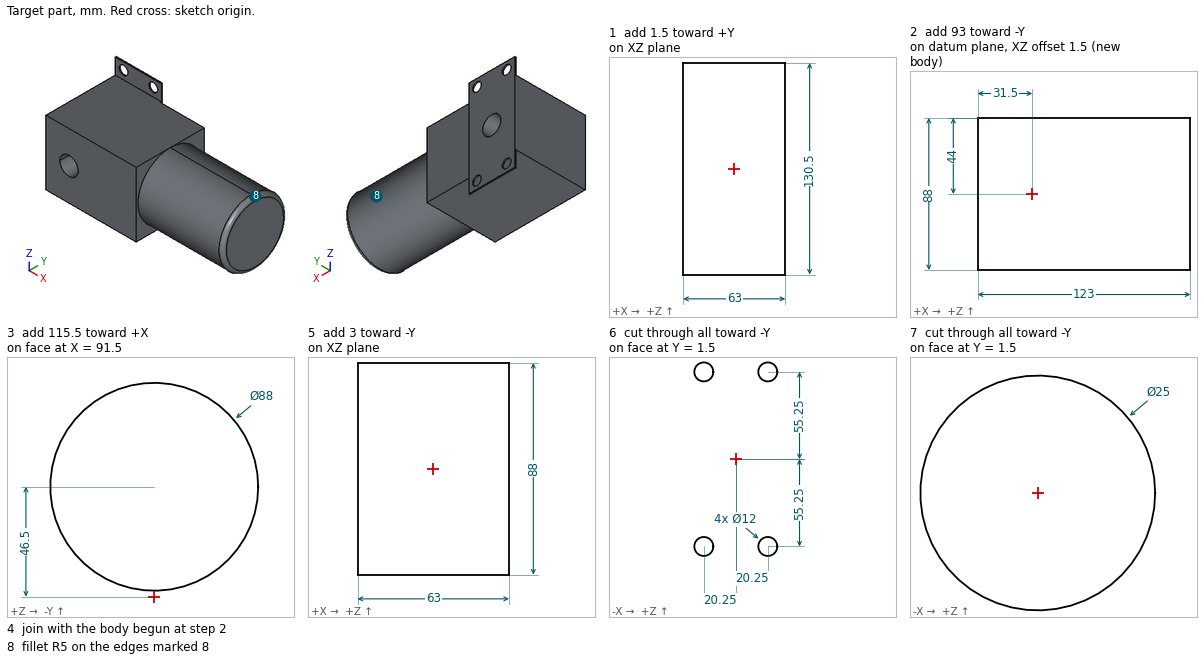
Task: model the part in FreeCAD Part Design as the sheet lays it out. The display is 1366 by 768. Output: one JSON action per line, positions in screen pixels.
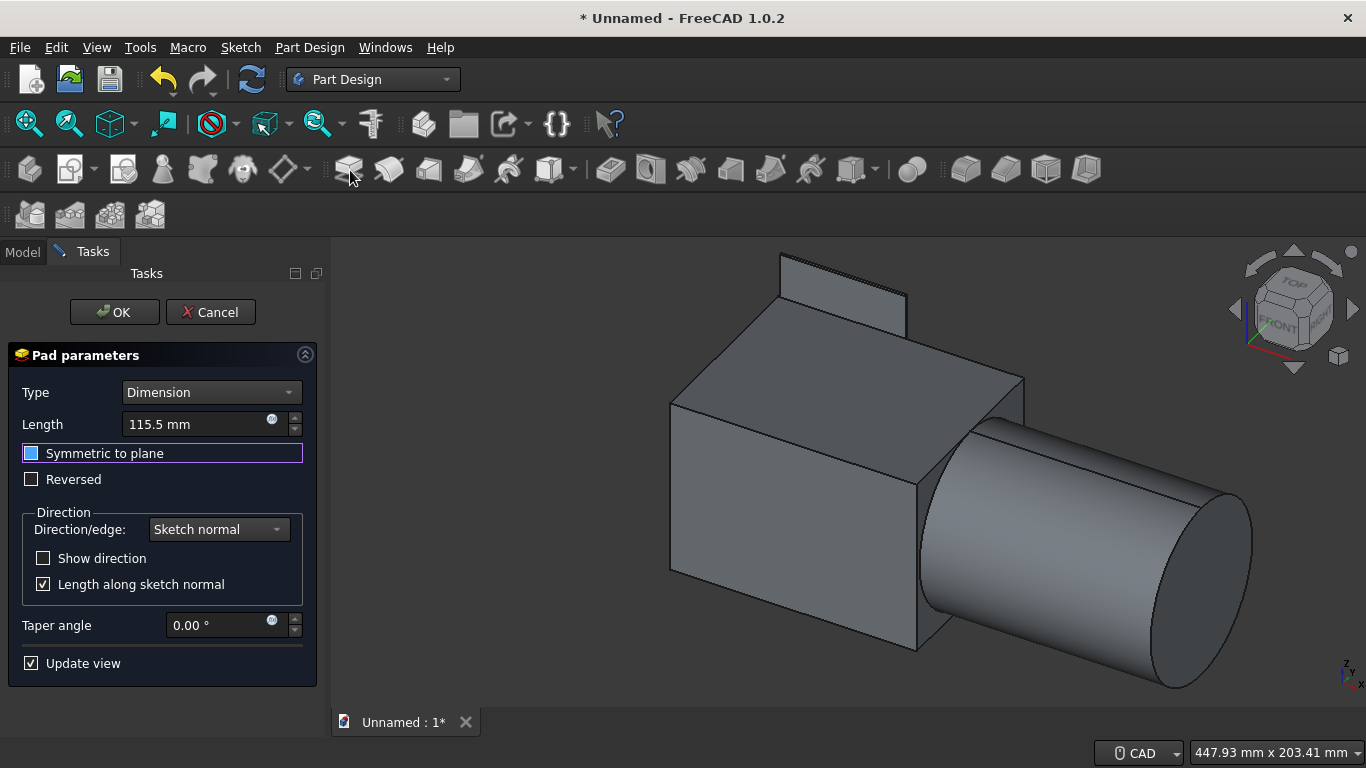
{"action": "left_click", "coordinate": [115, 312]}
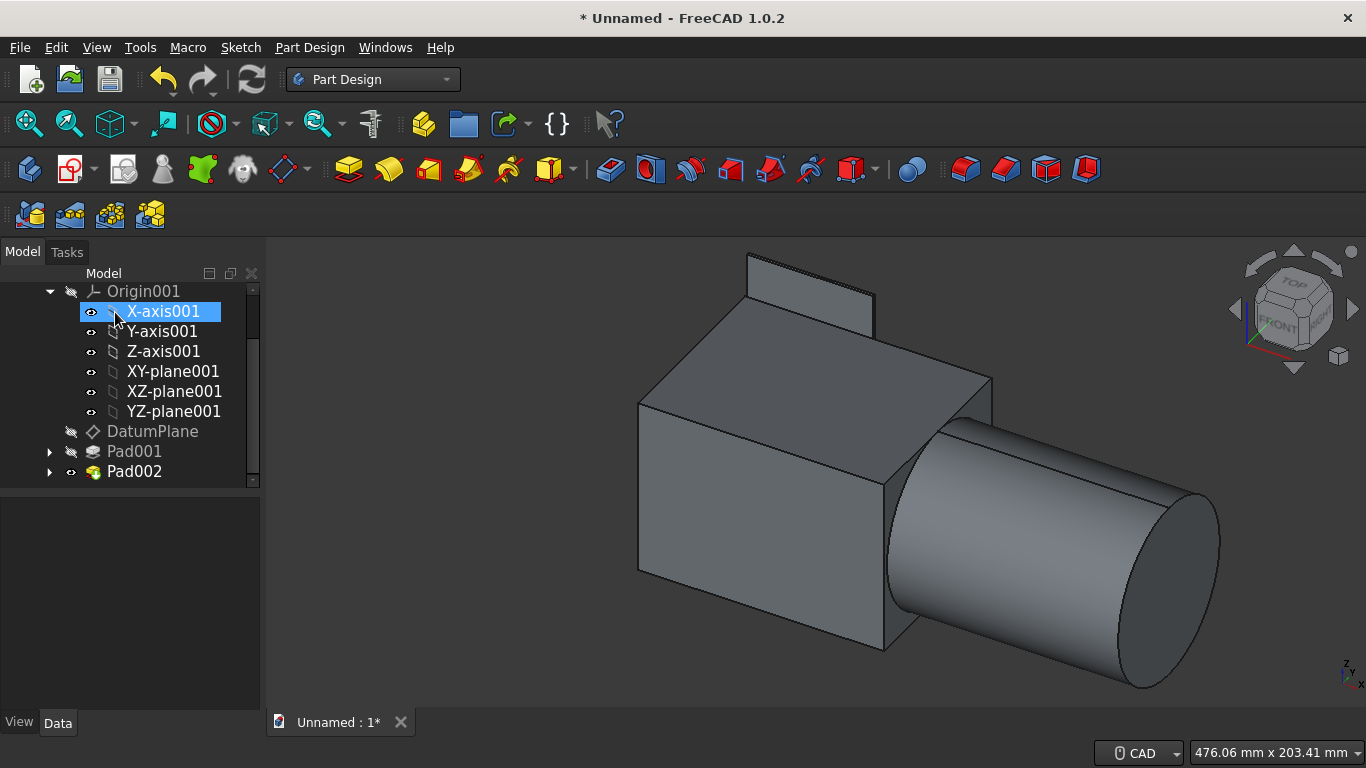
{"action": "left_click", "coordinate": [30, 124]}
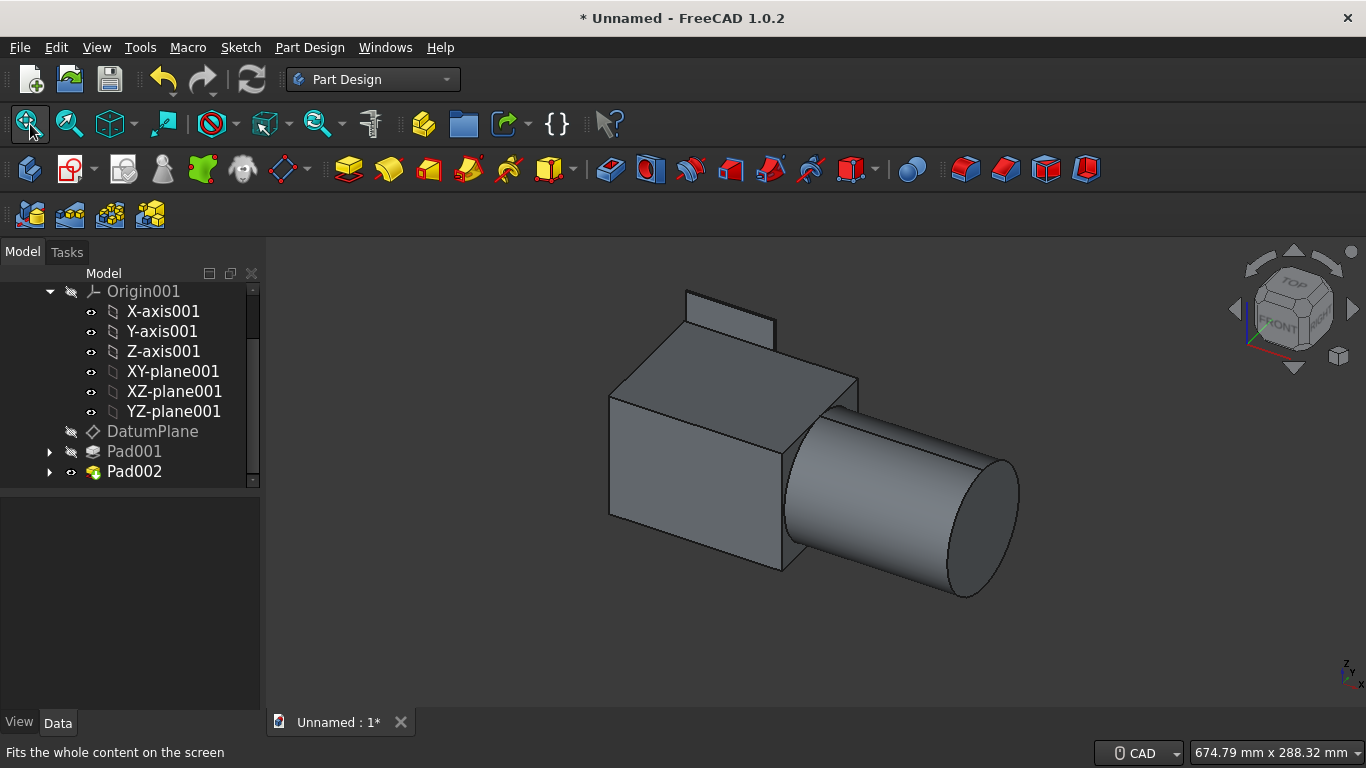
{"action": "scroll", "coordinate": [140, 387], "scroll_direction": "down", "scroll_amount": 3}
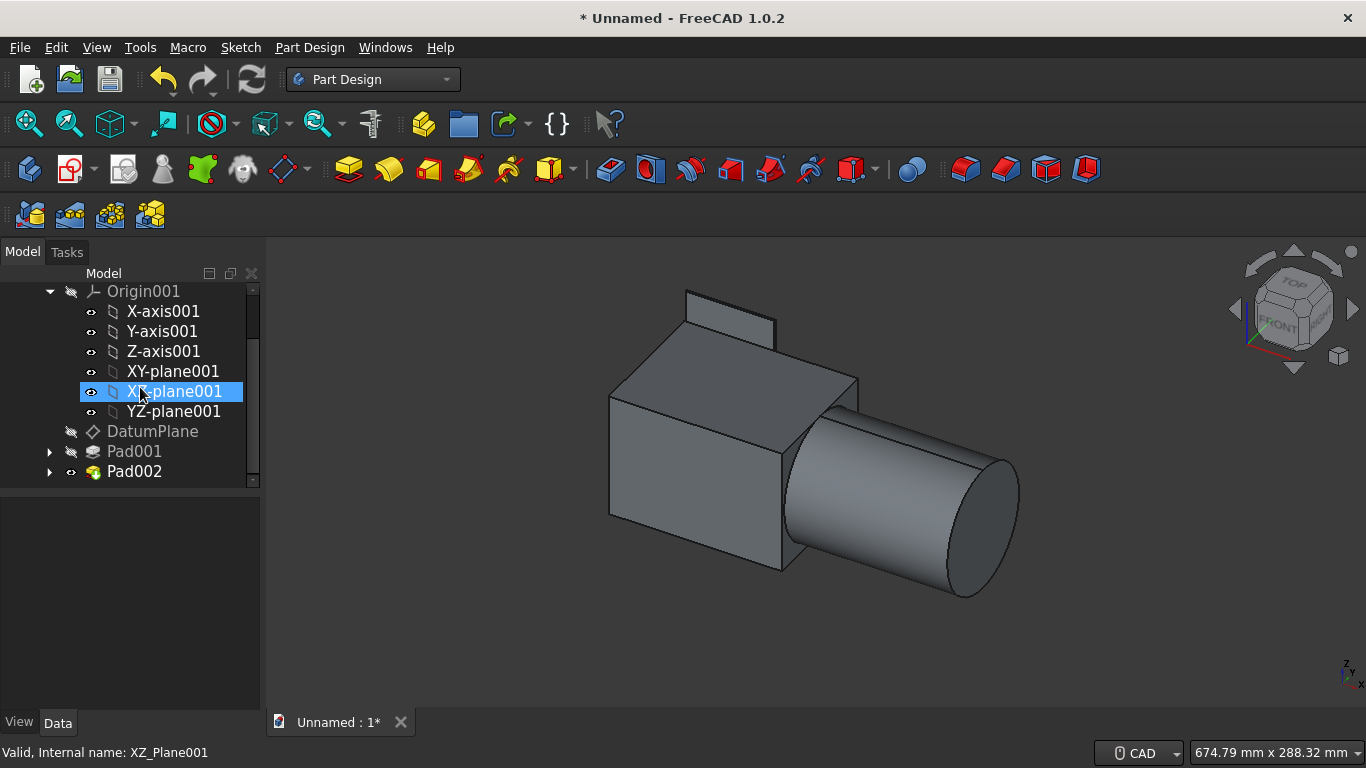
{"action": "scroll", "coordinate": [140, 387], "scroll_direction": "up", "scroll_amount": 15}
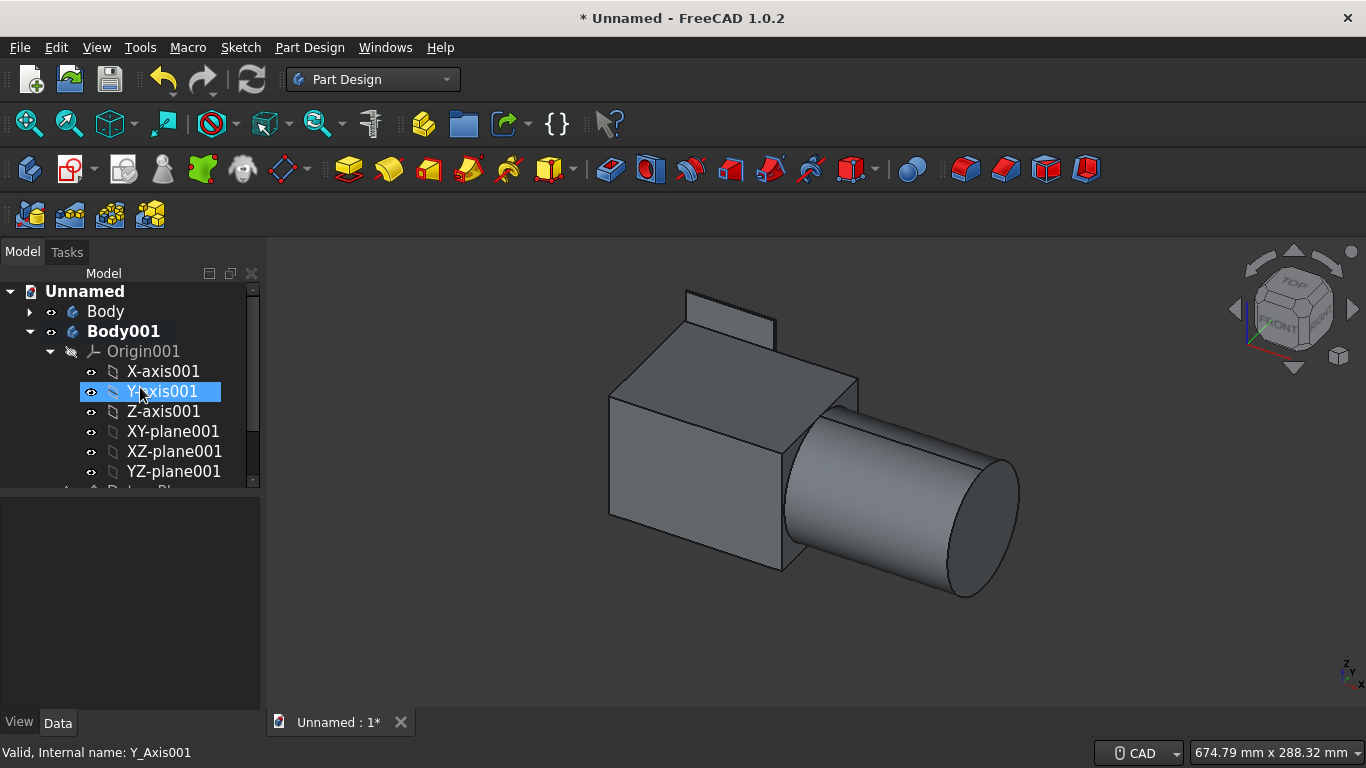
{"action": "double_click", "coordinate": [96, 312]}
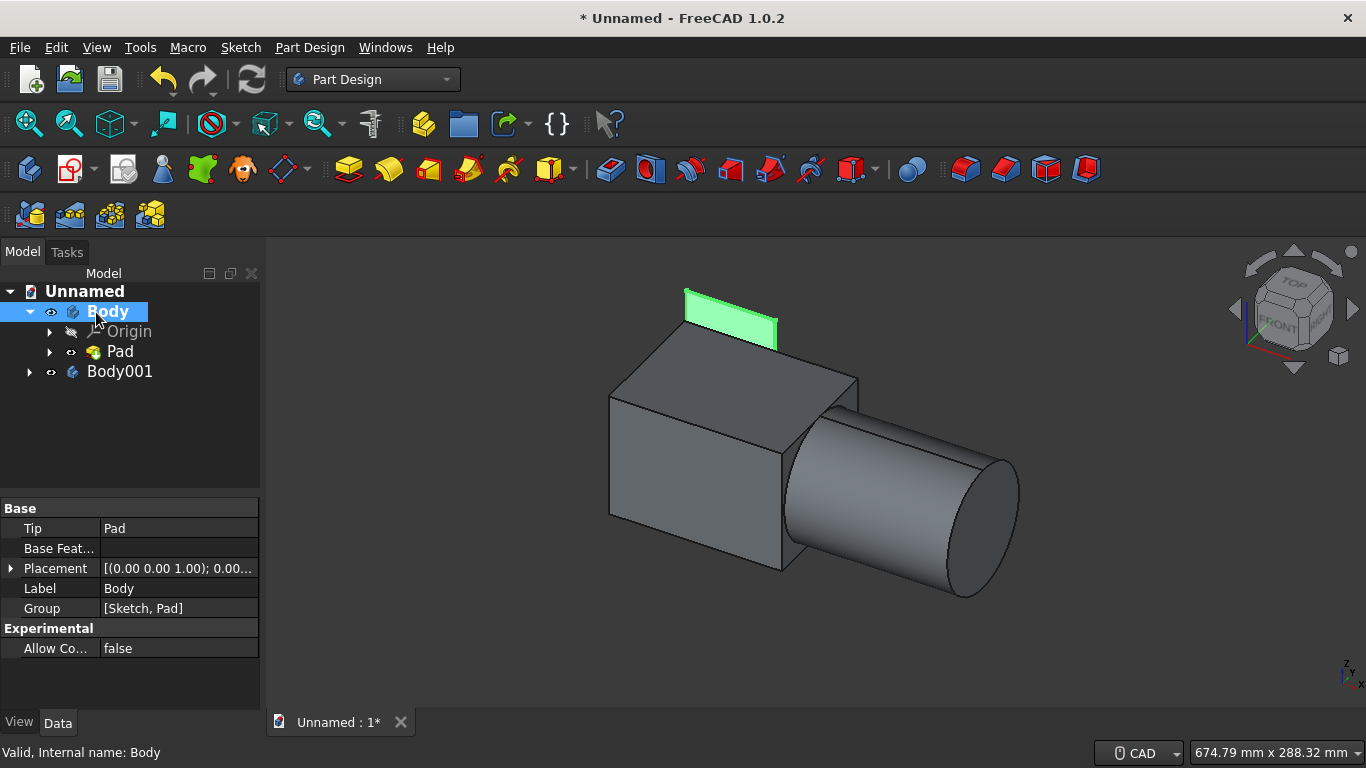
{"action": "left_click", "coordinate": [96, 312]}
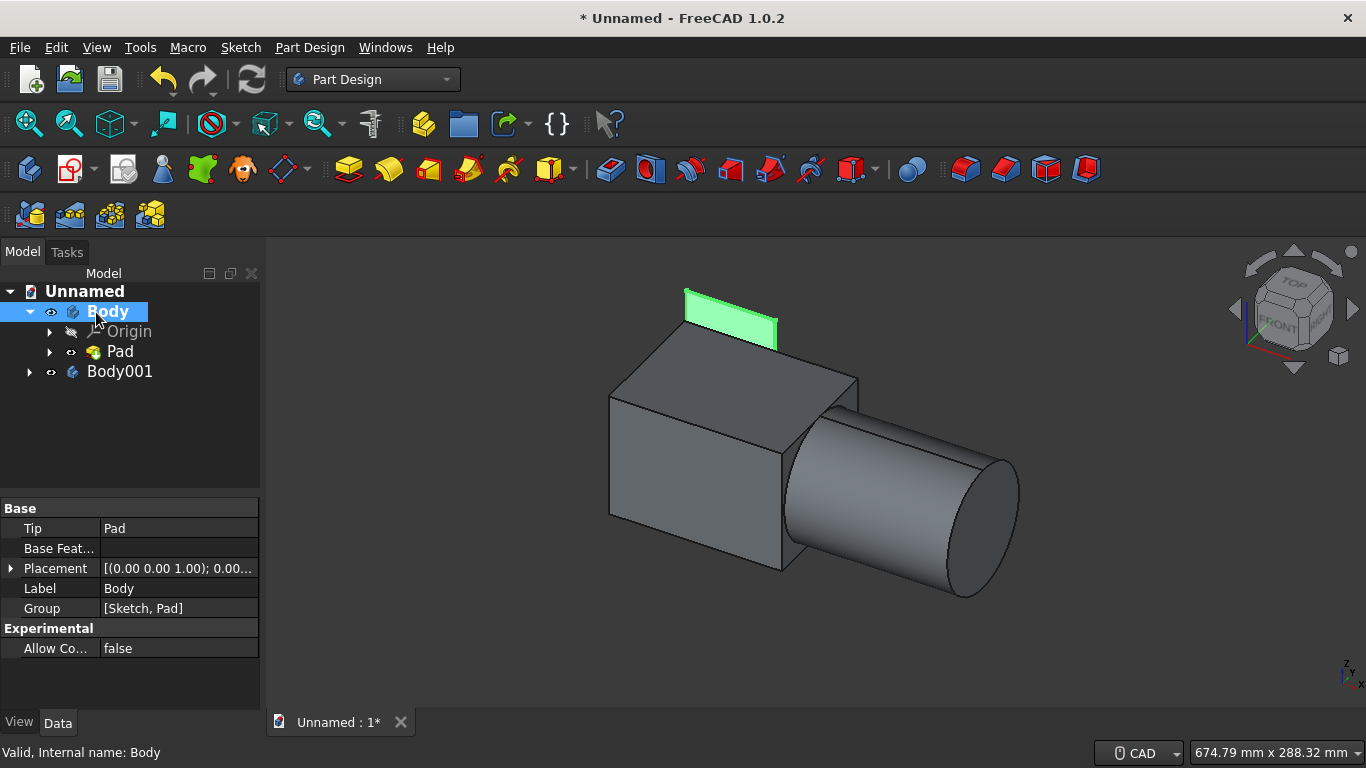
{"action": "left_click", "coordinate": [146, 648]}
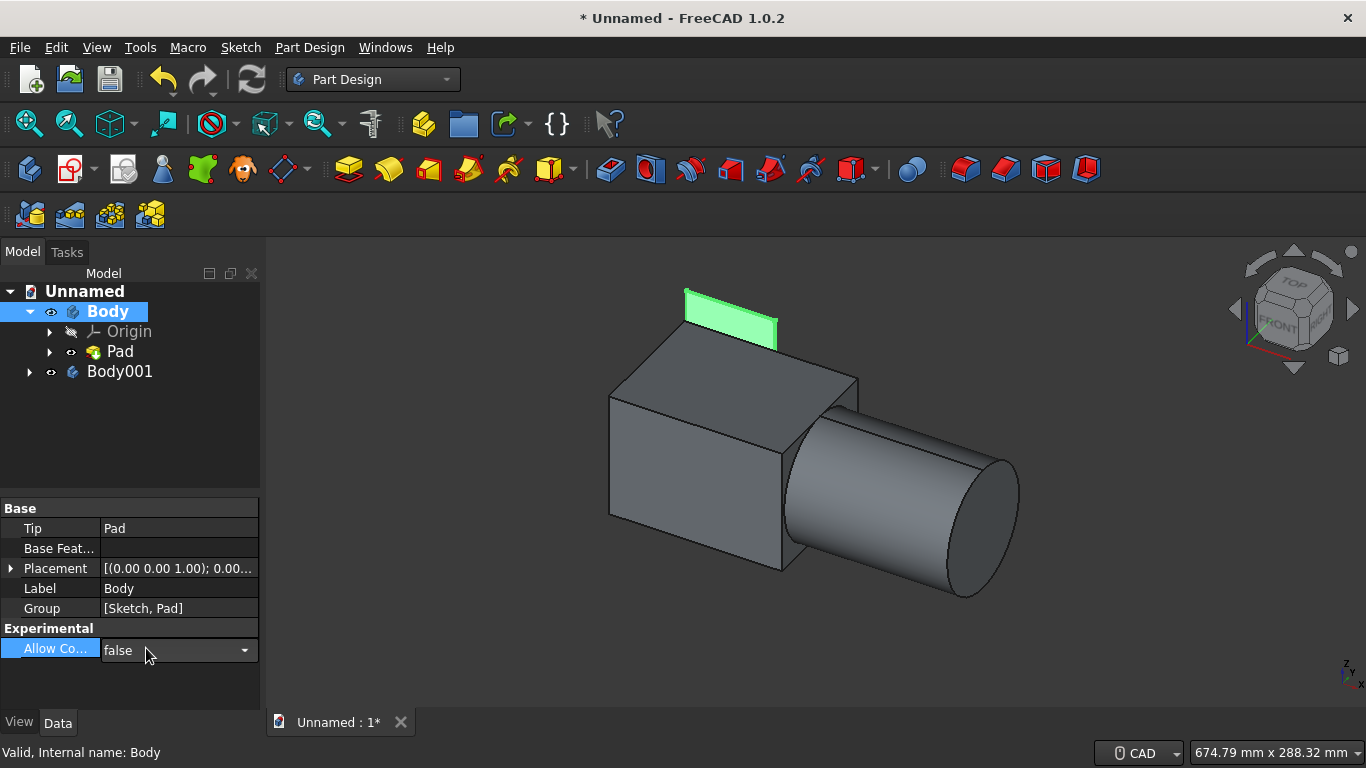
{"action": "left_click", "coordinate": [146, 648]}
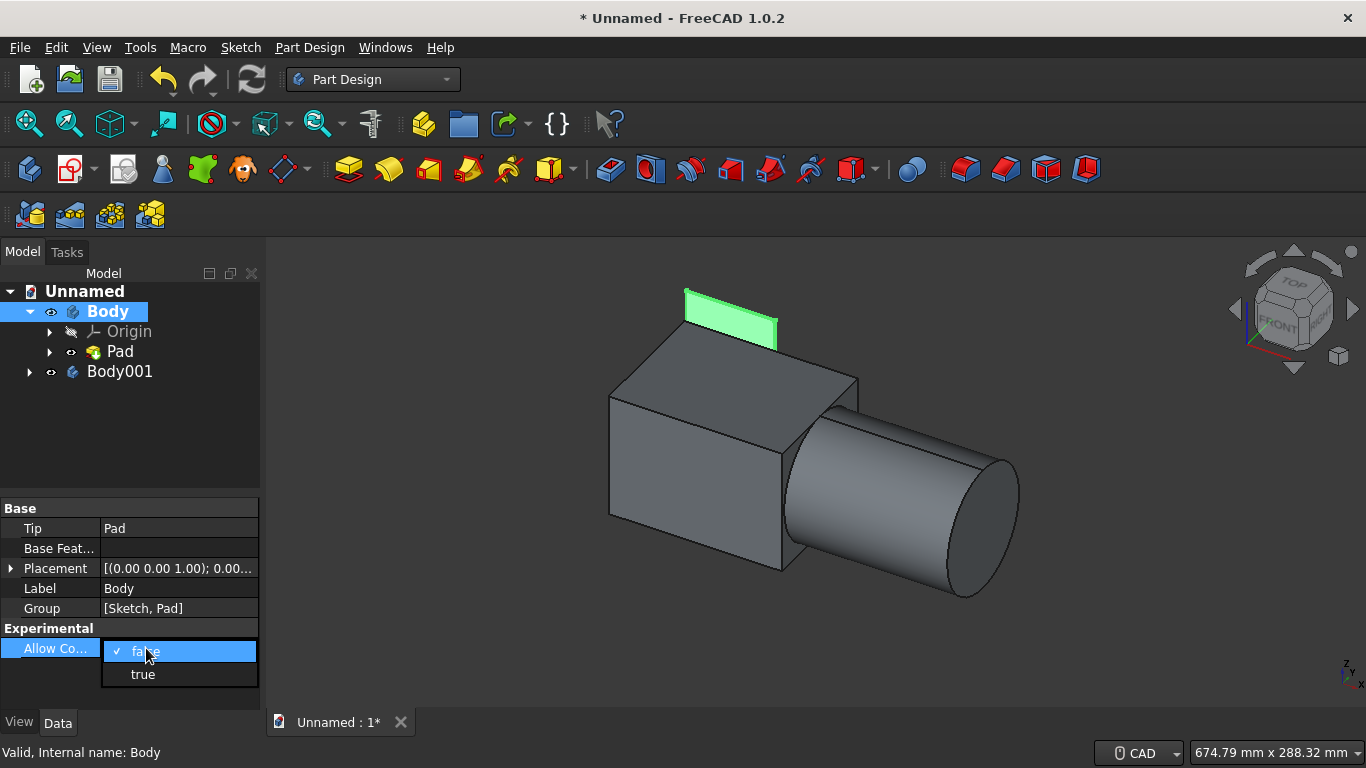
{"action": "left_click", "coordinate": [179, 674]}
{"action": "key", "text": "Return"}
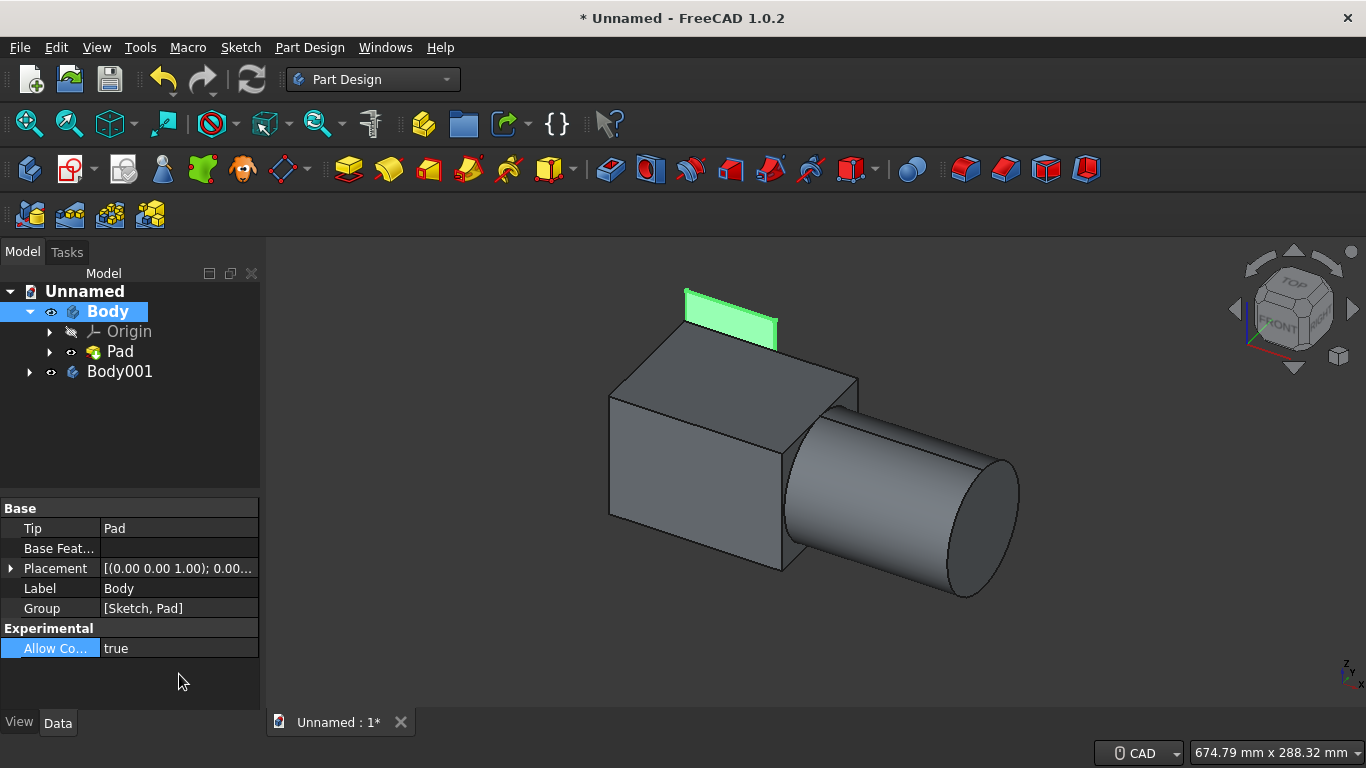
{"action": "left_click", "coordinate": [96, 372]}